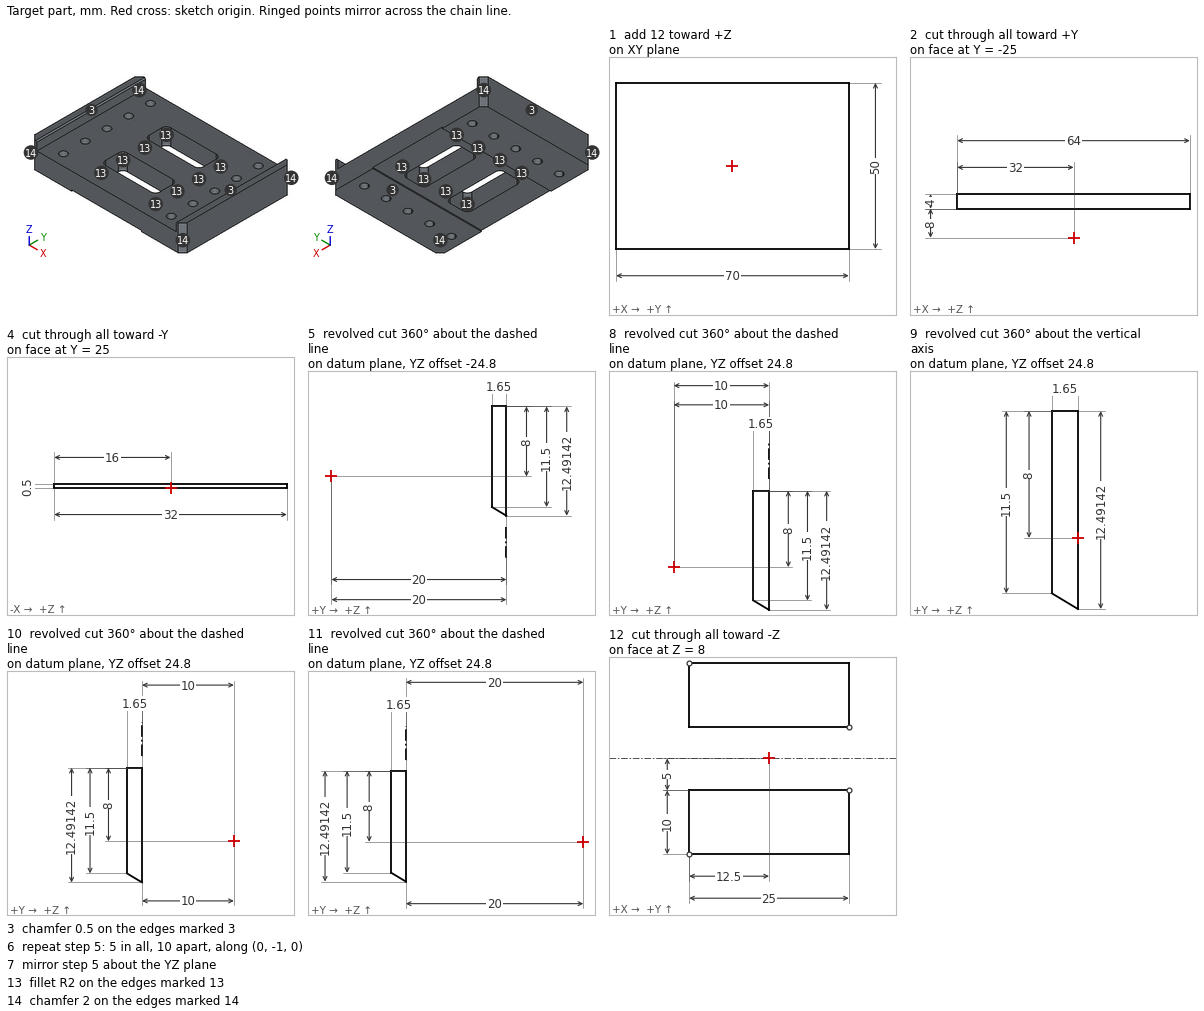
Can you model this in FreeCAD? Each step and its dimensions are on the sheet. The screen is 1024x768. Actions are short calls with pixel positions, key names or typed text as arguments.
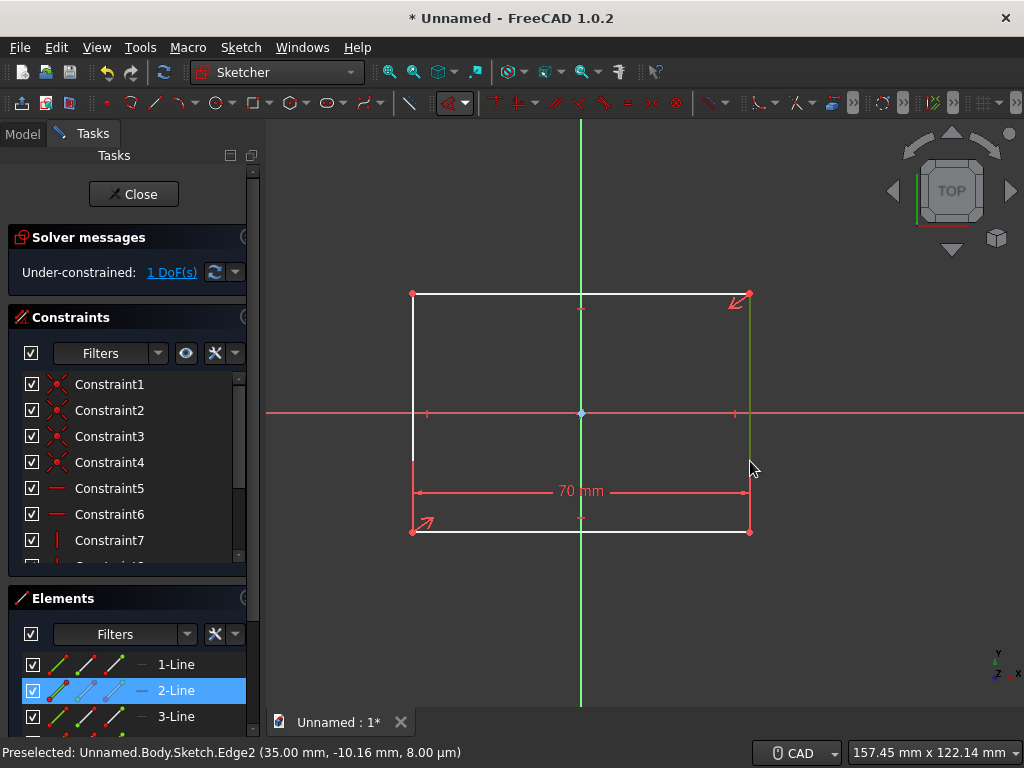
key(i)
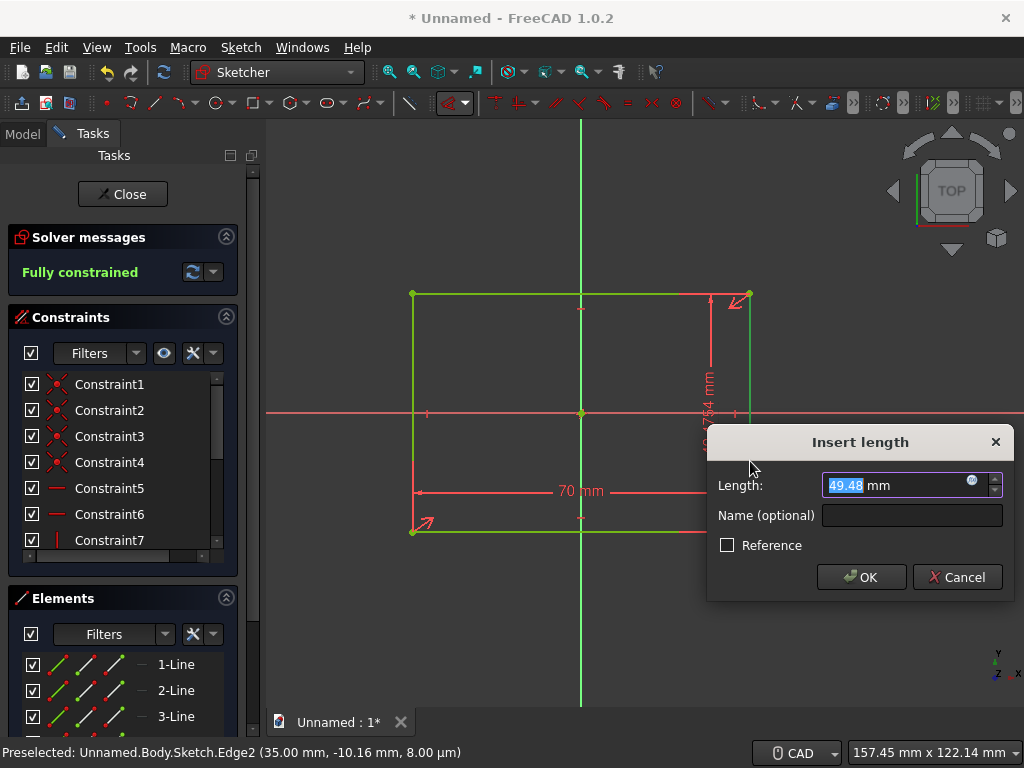
text(50)
key(Return)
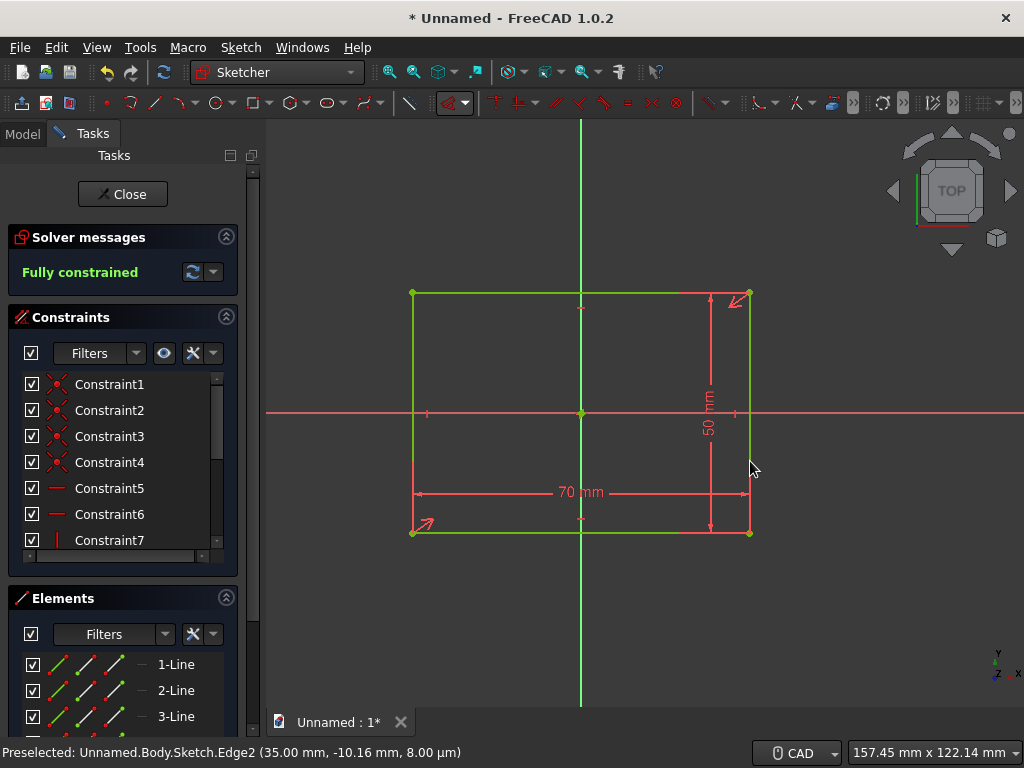
click(123, 194)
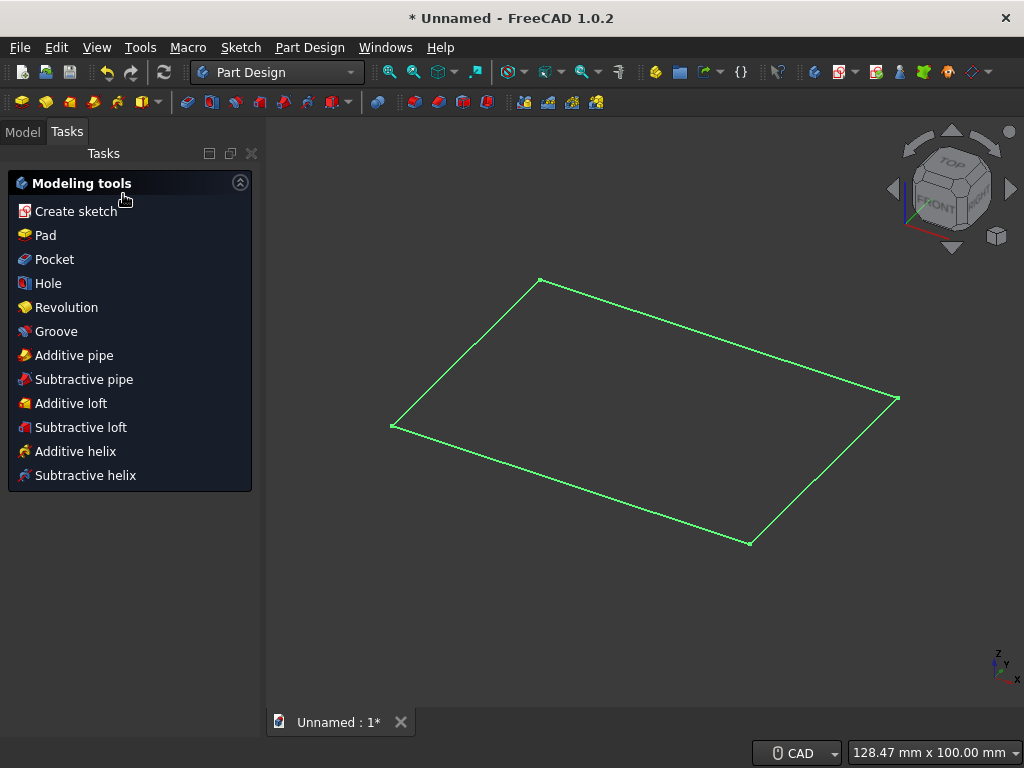
click(22, 102)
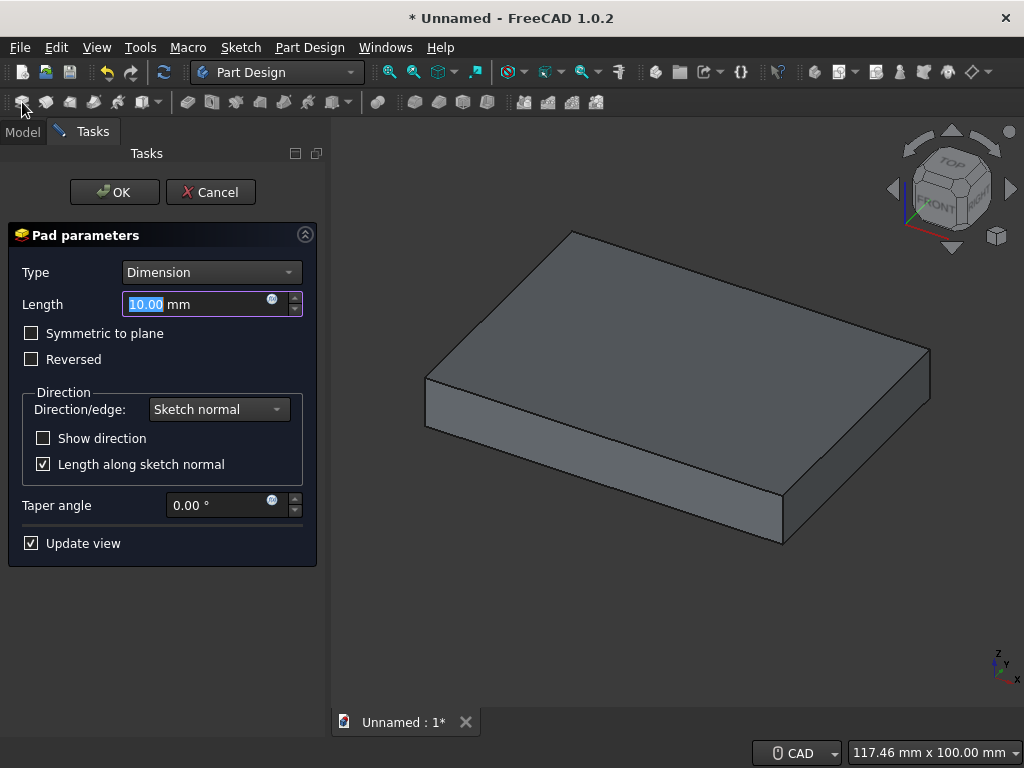
text(12)
key(Tab)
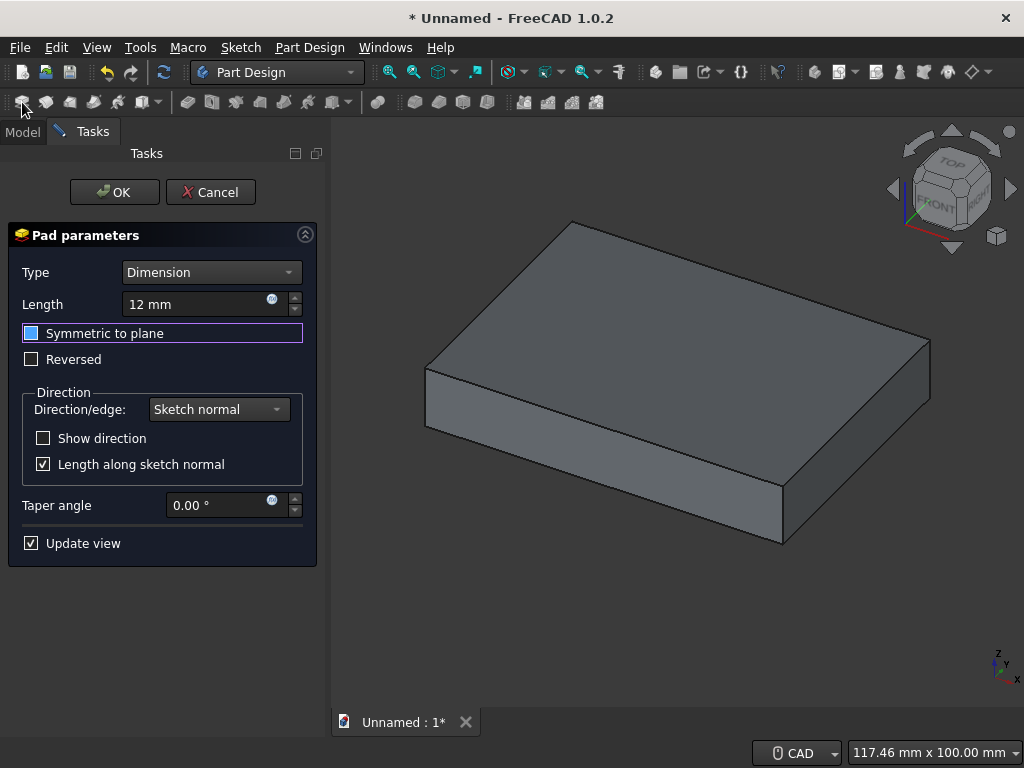
click(115, 192)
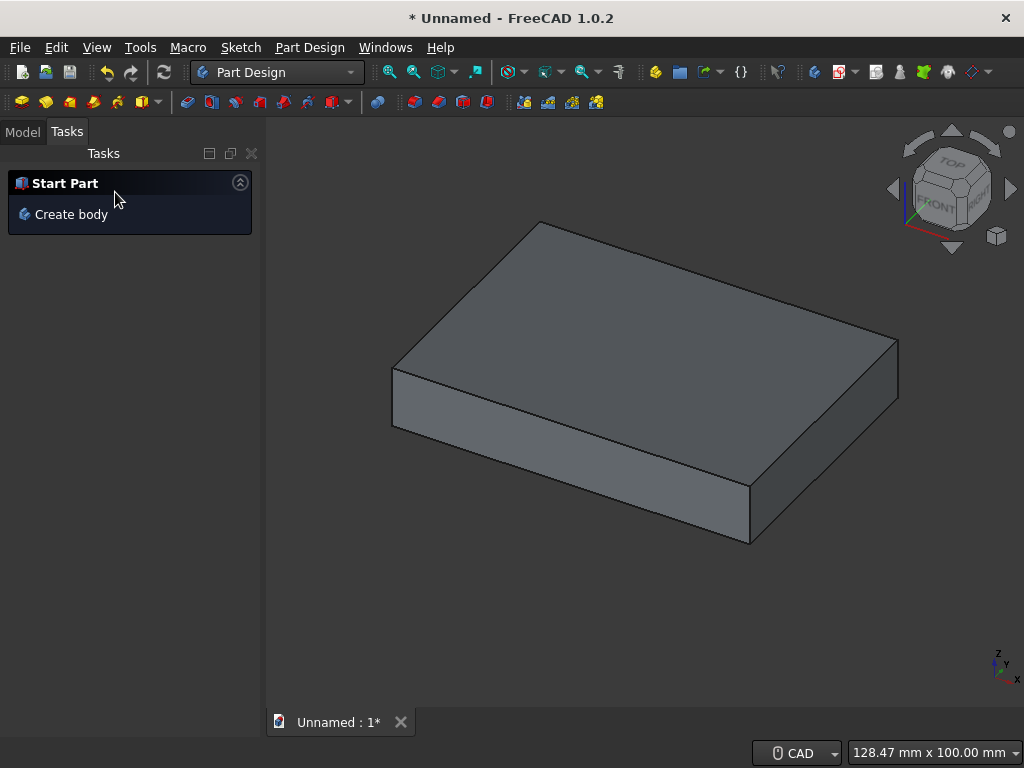
click(673, 489)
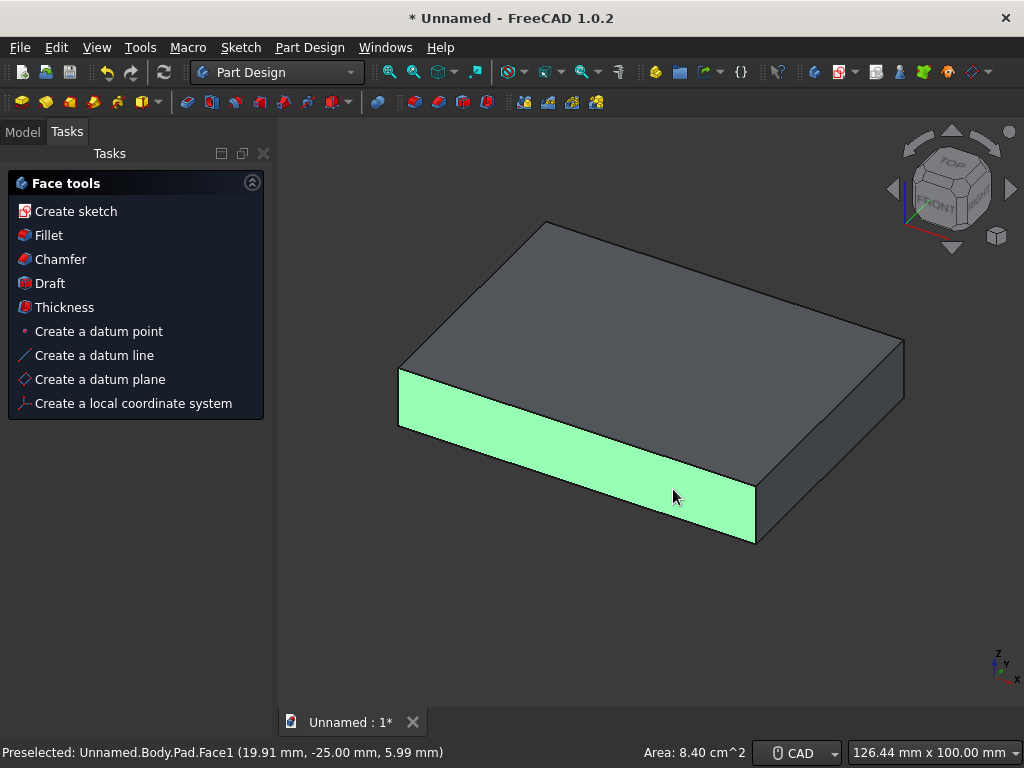
click(840, 72)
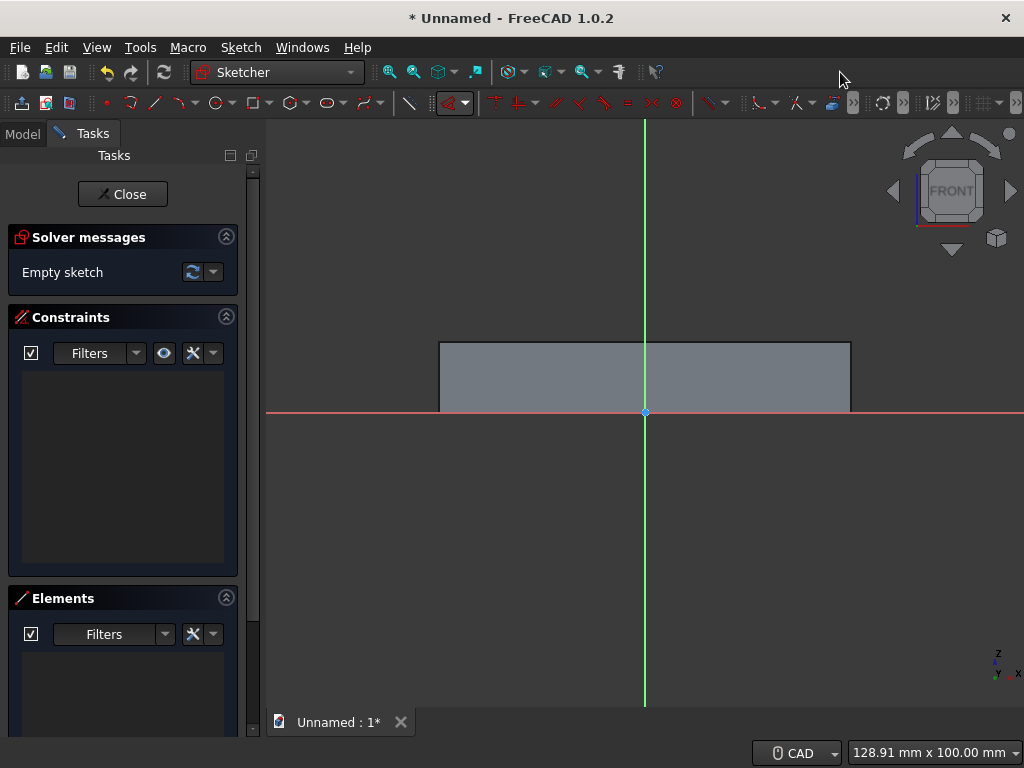
key(g)
key(r)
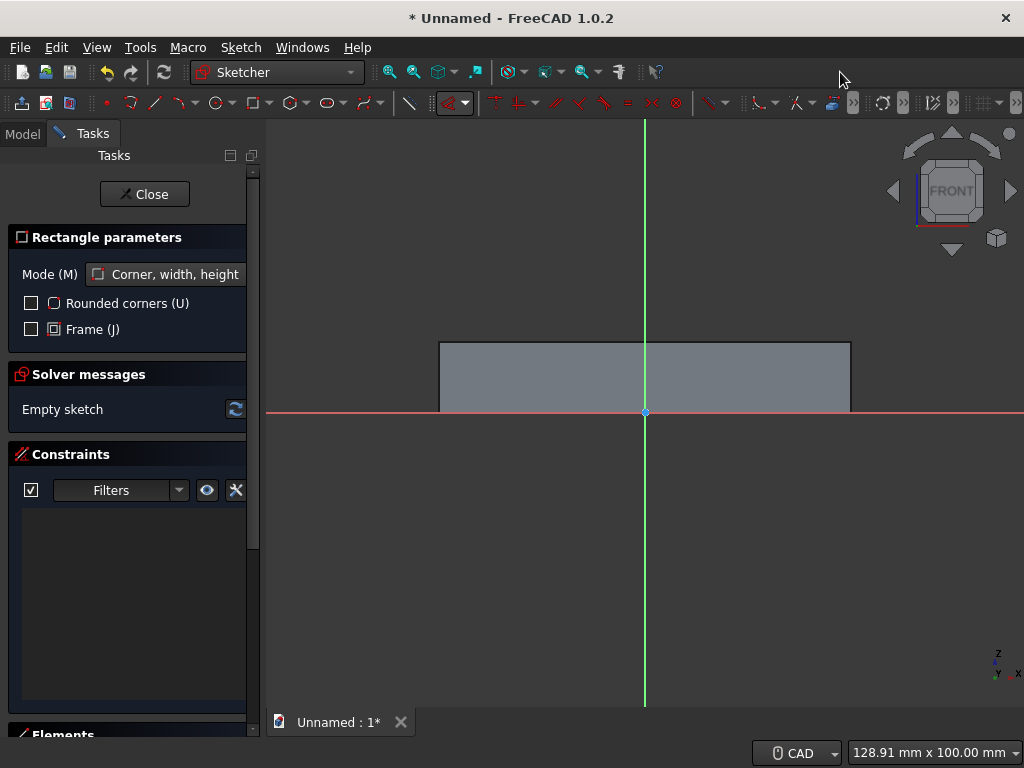
click(457, 342)
click(833, 366)
key(Escape)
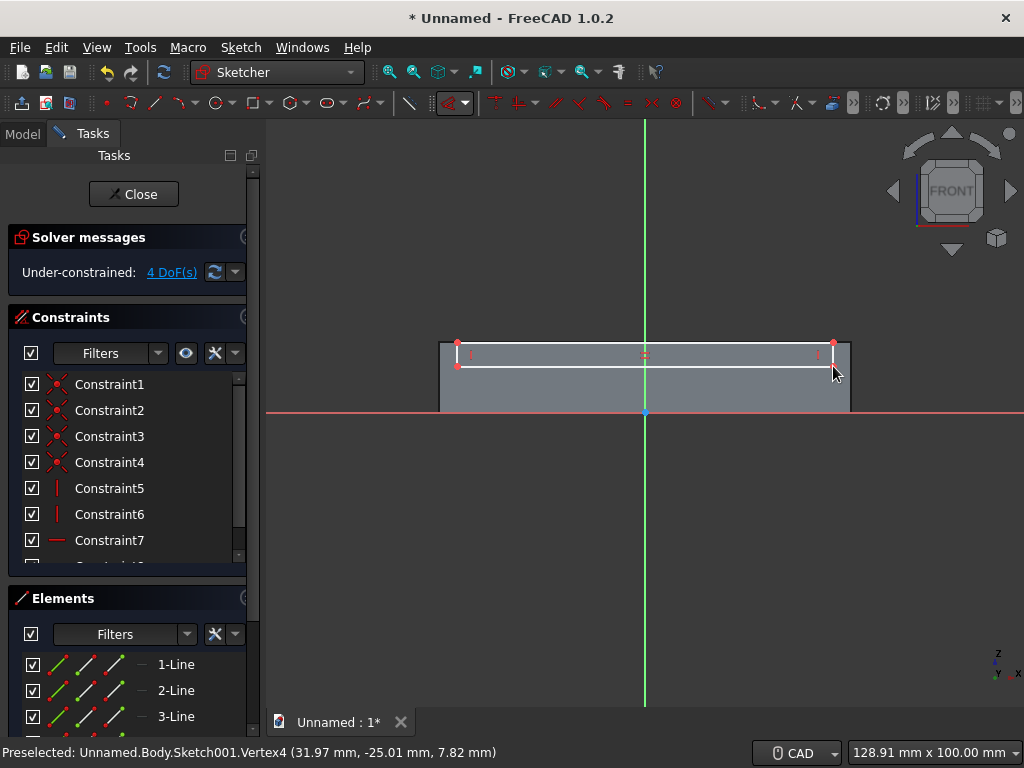
scroll(457, 353, up, 3)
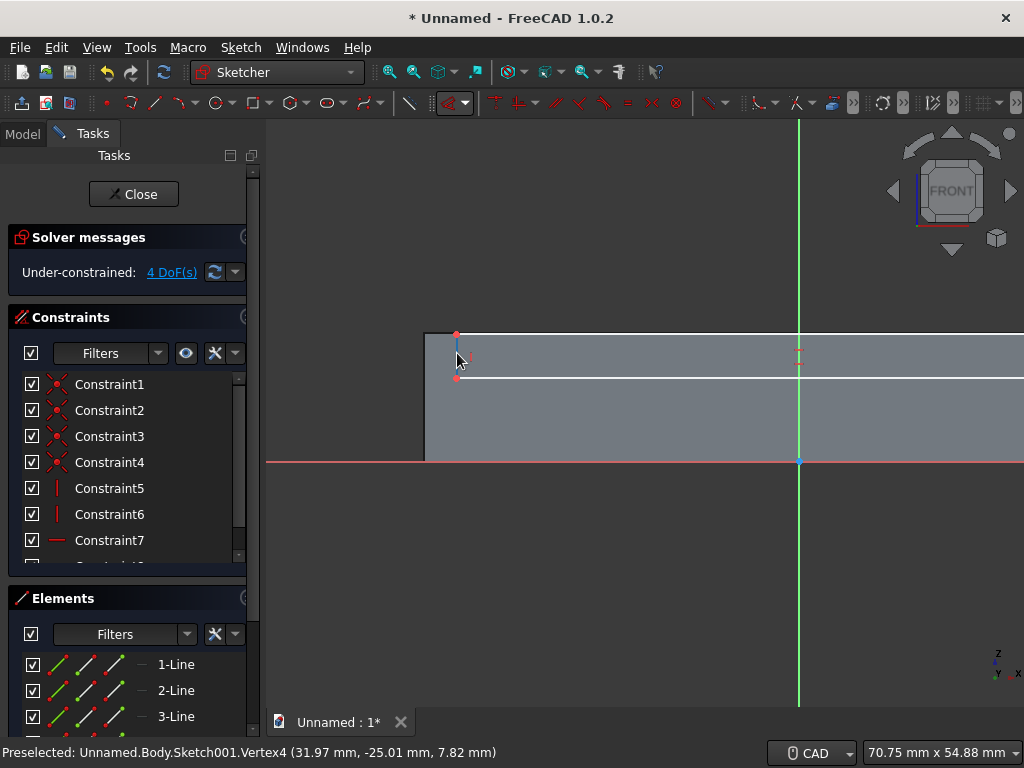
click(457, 352)